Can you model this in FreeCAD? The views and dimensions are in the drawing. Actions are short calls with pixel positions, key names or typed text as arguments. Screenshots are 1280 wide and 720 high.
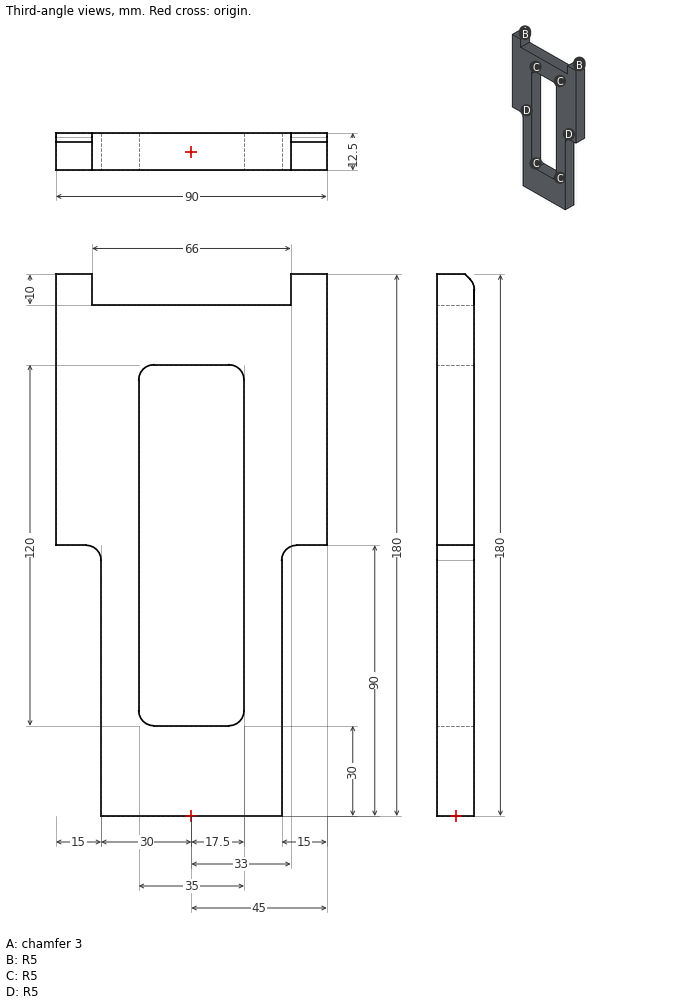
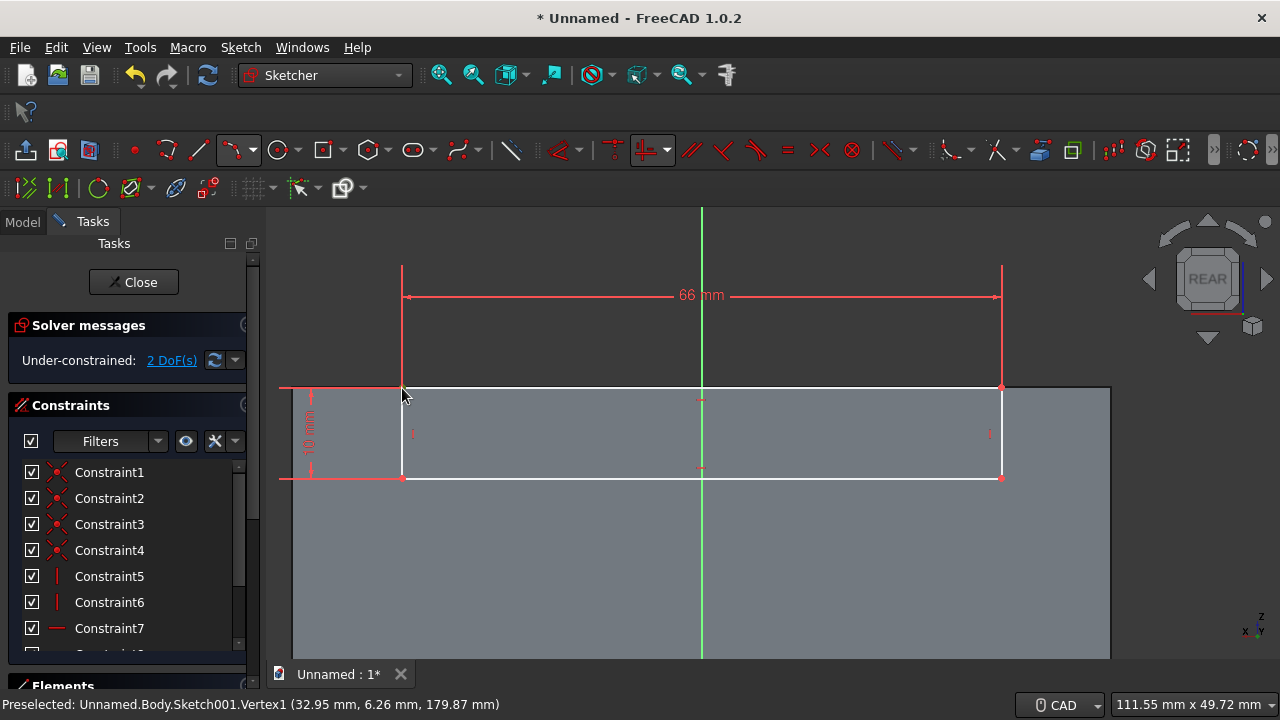
click(582, 150)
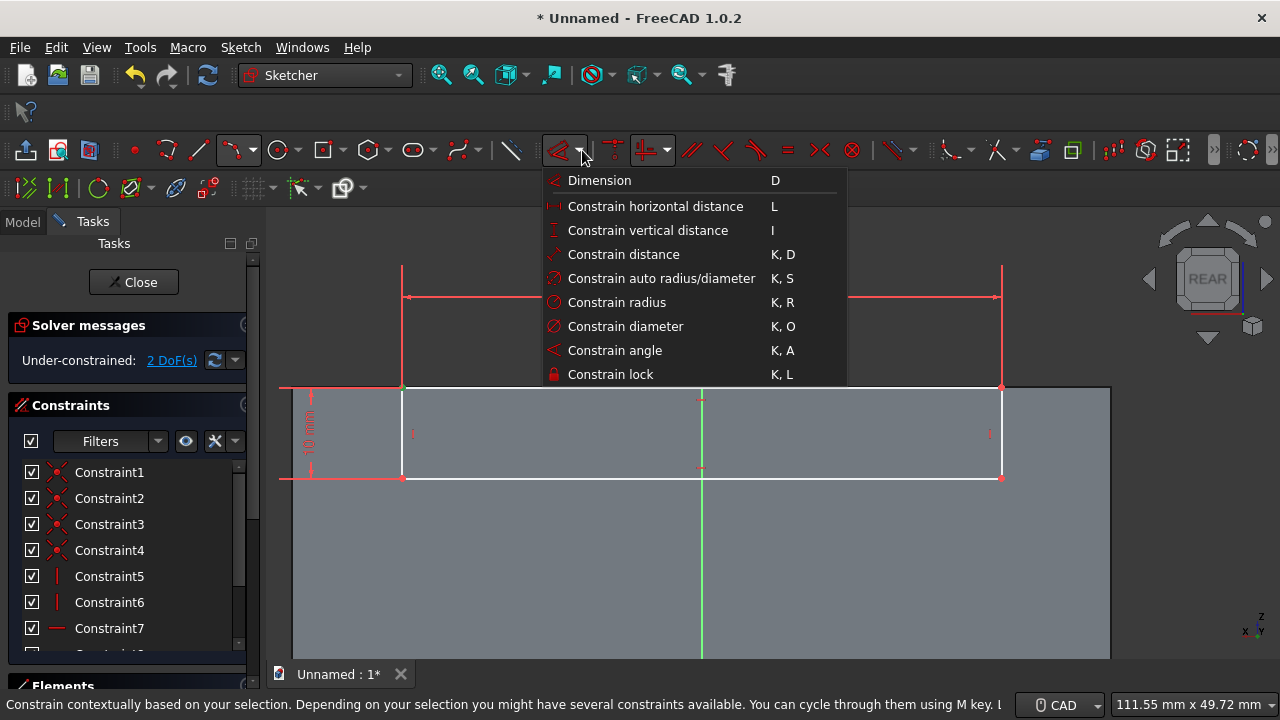
click(695, 206)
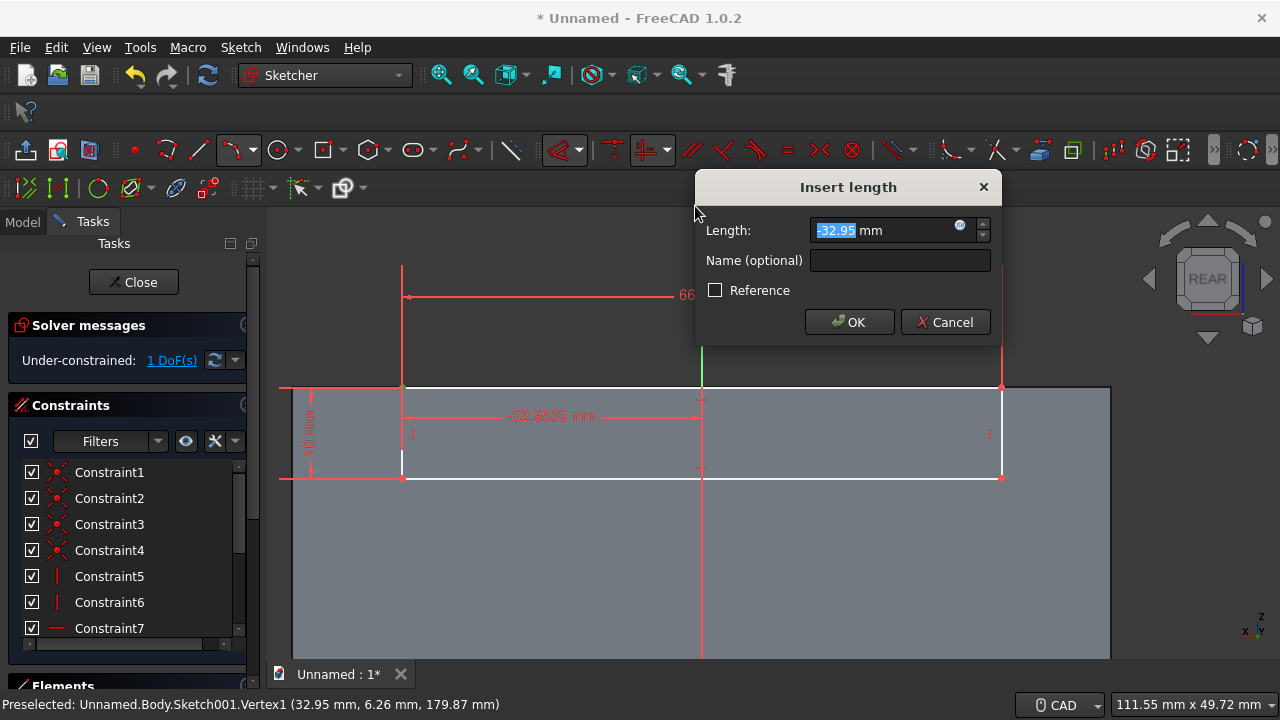
text(-33)
key(Return)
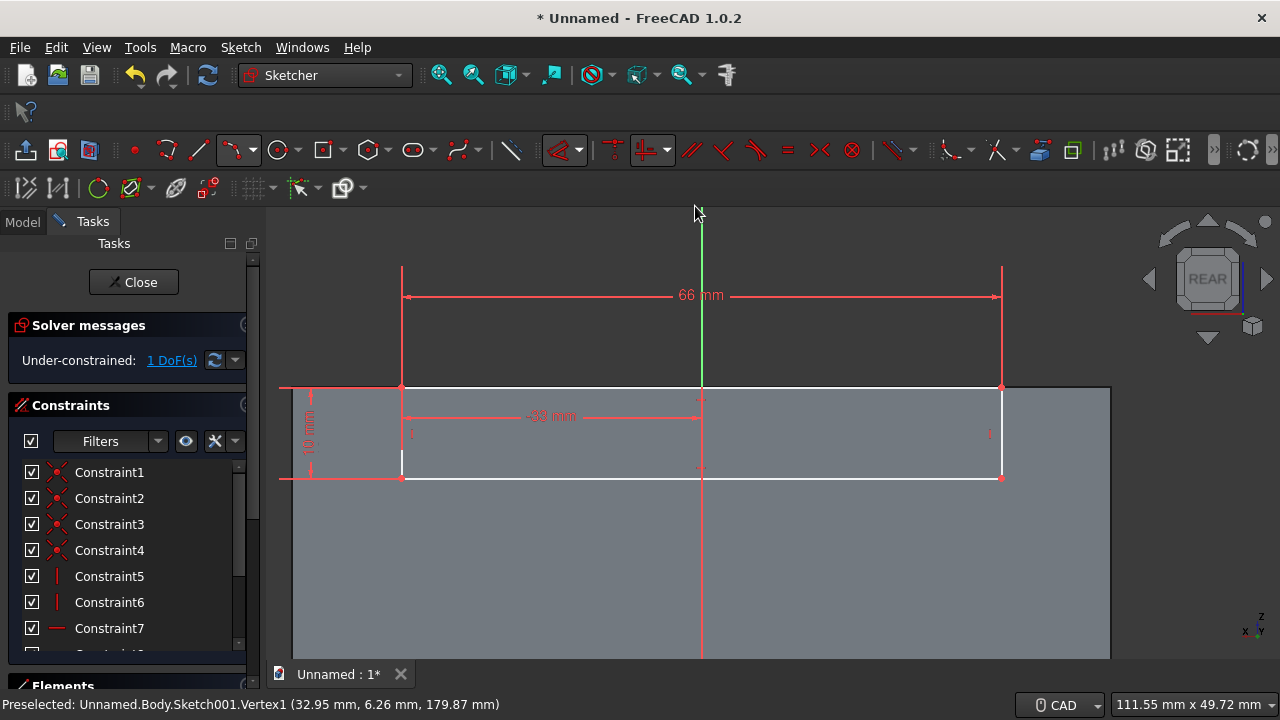
click(402, 388)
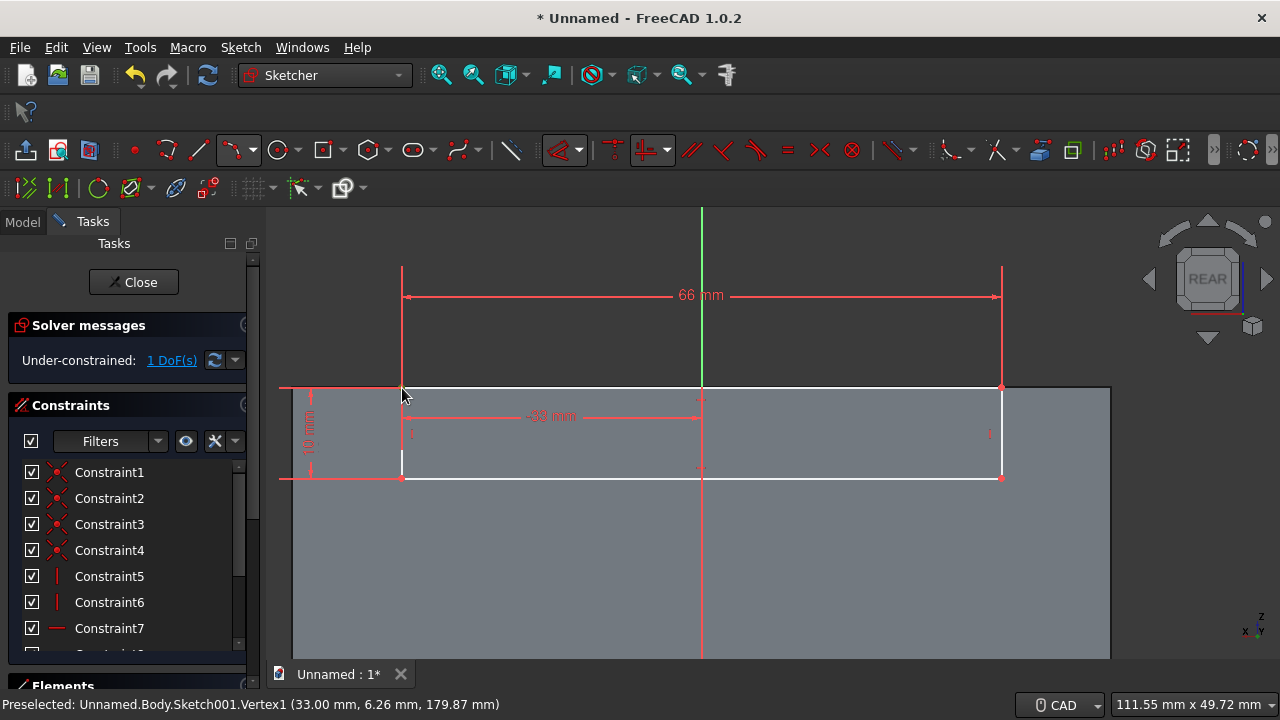
click(582, 150)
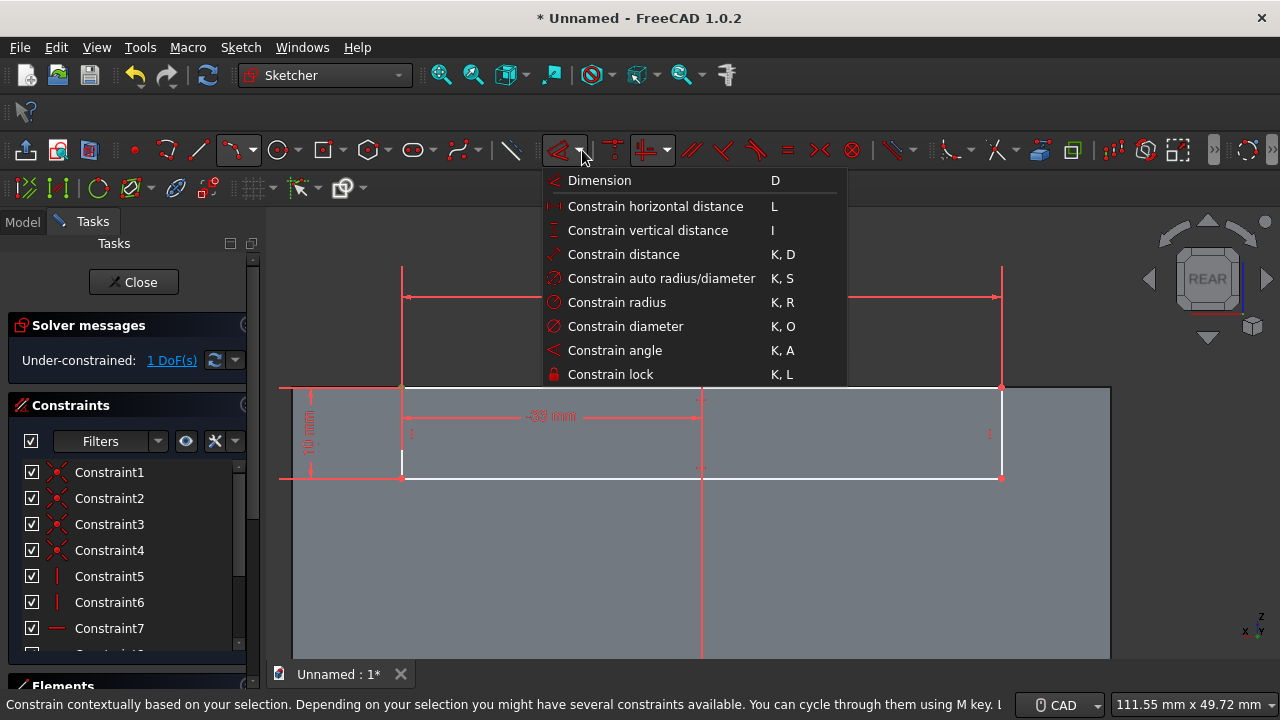
click(695, 230)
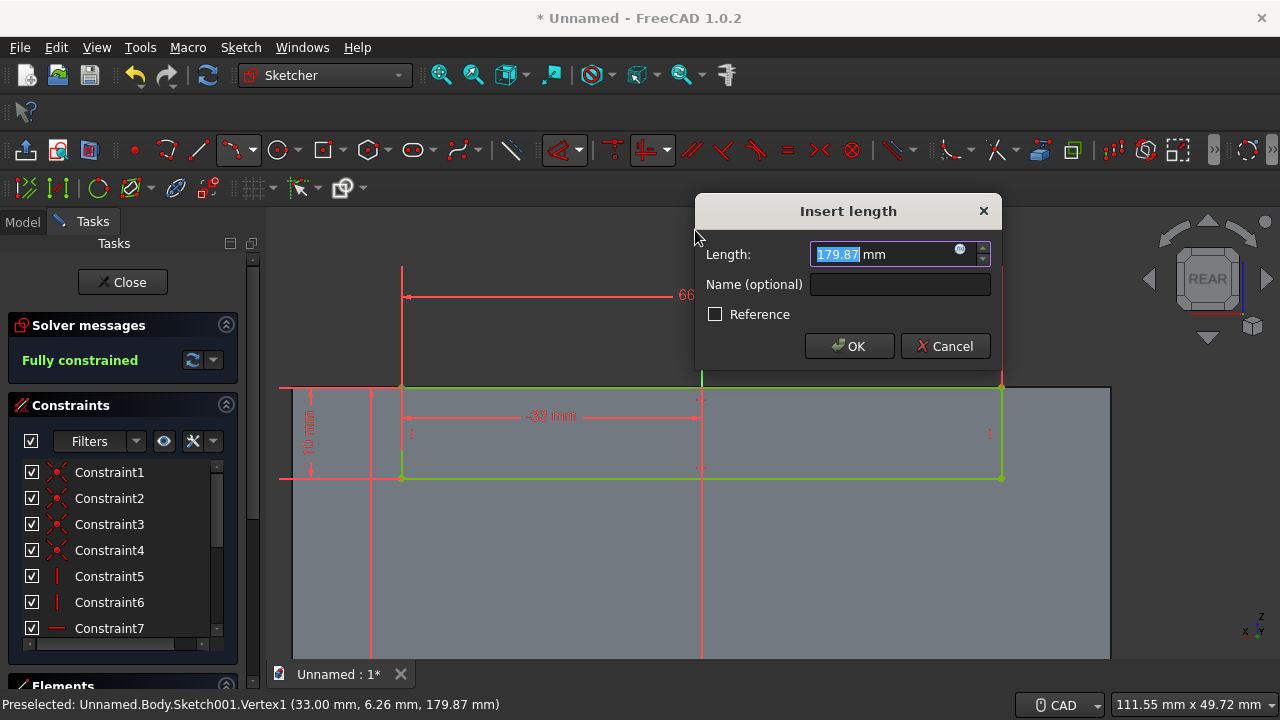
text(180)
key(Return)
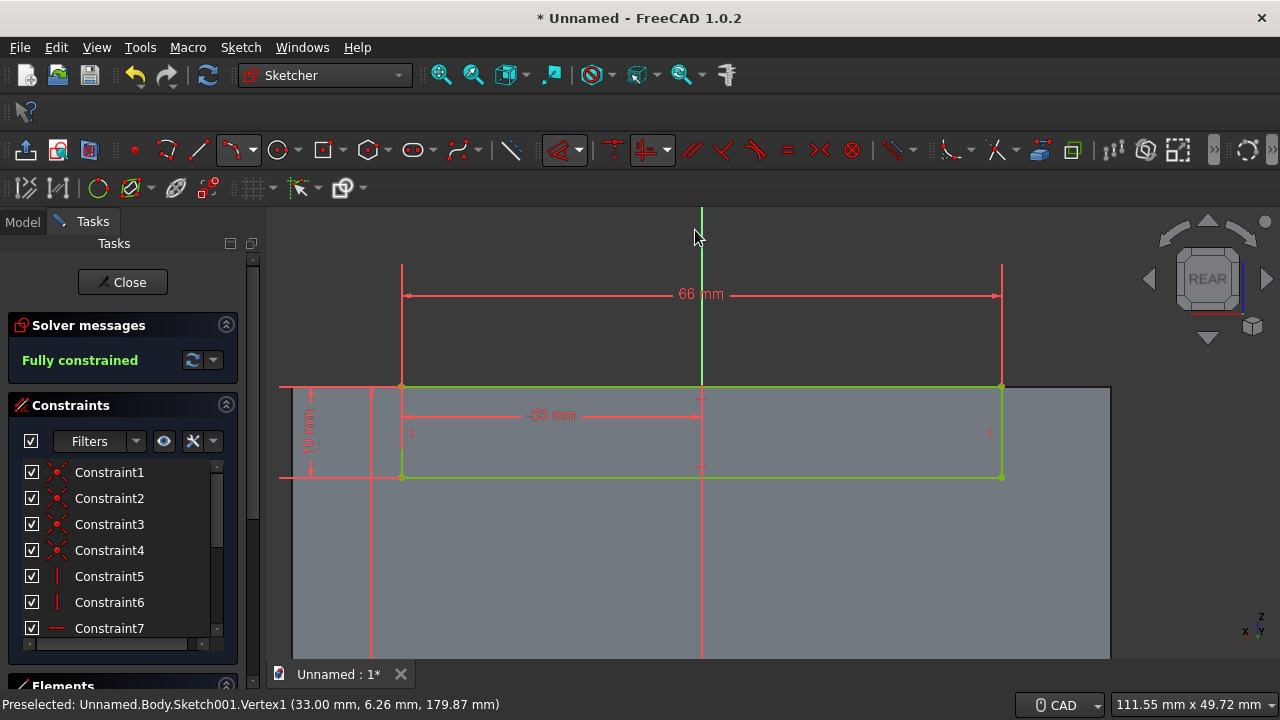
click(123, 282)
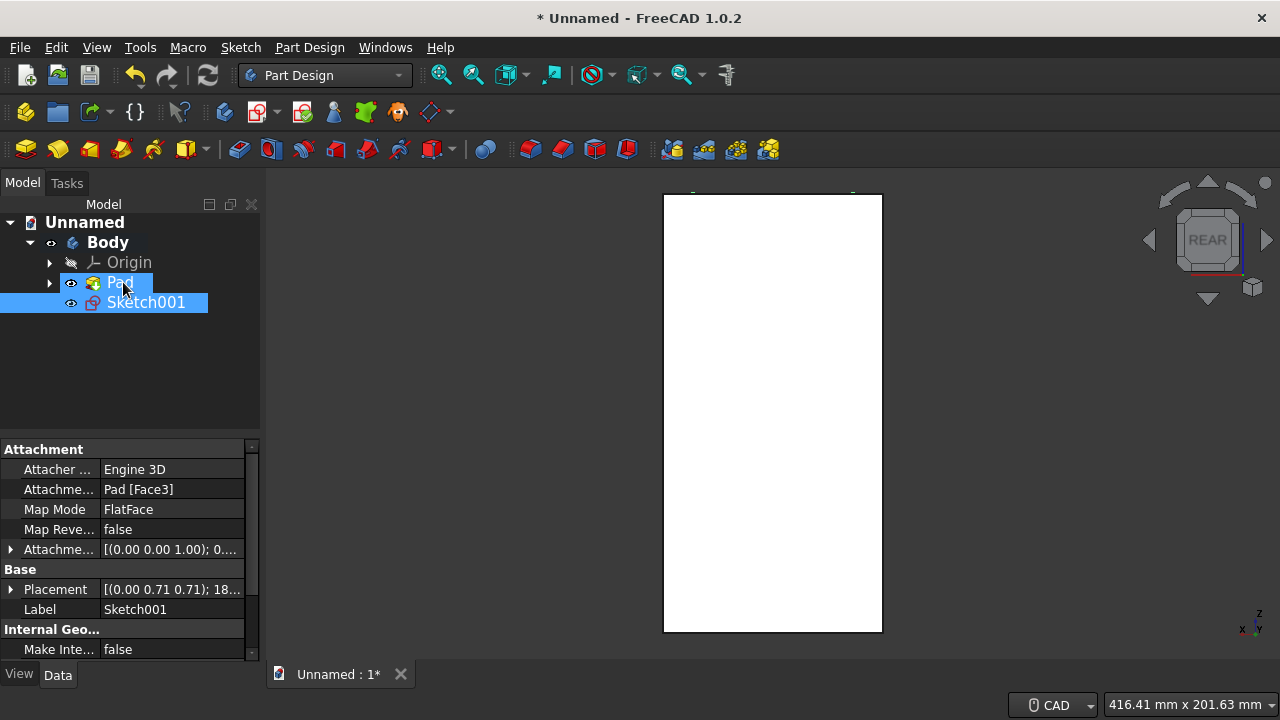
click(240, 150)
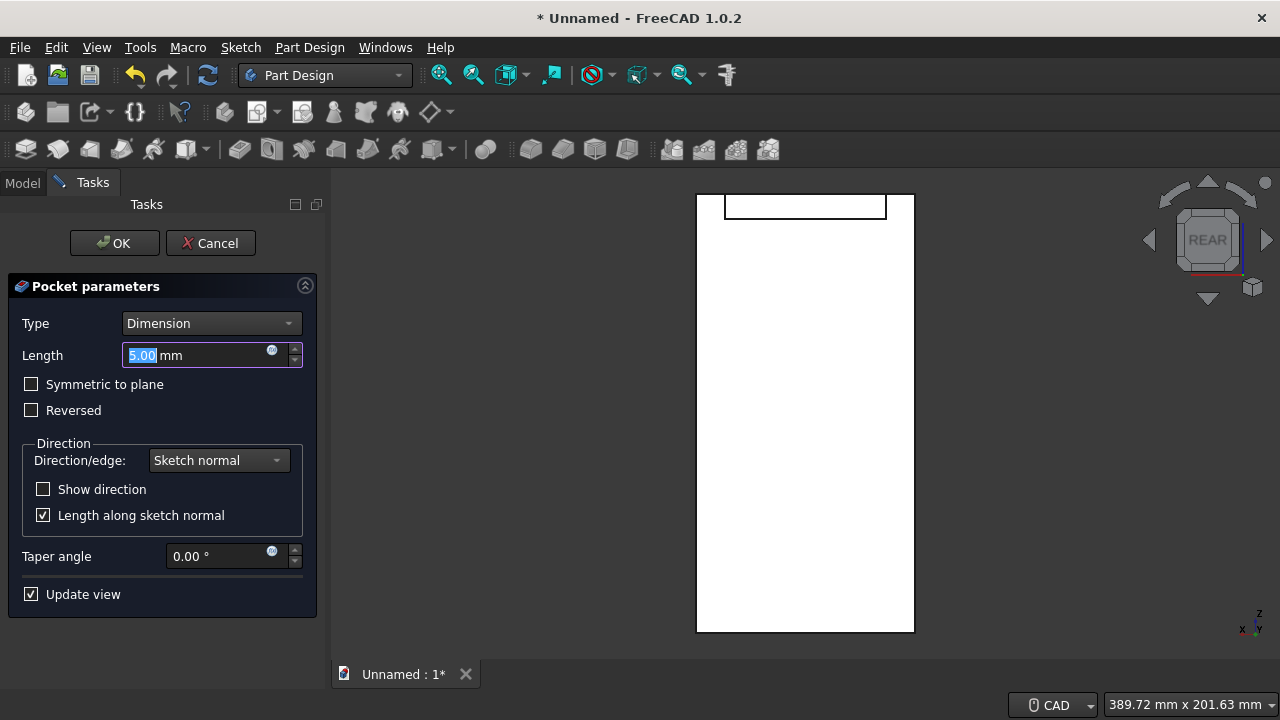
click(212, 324)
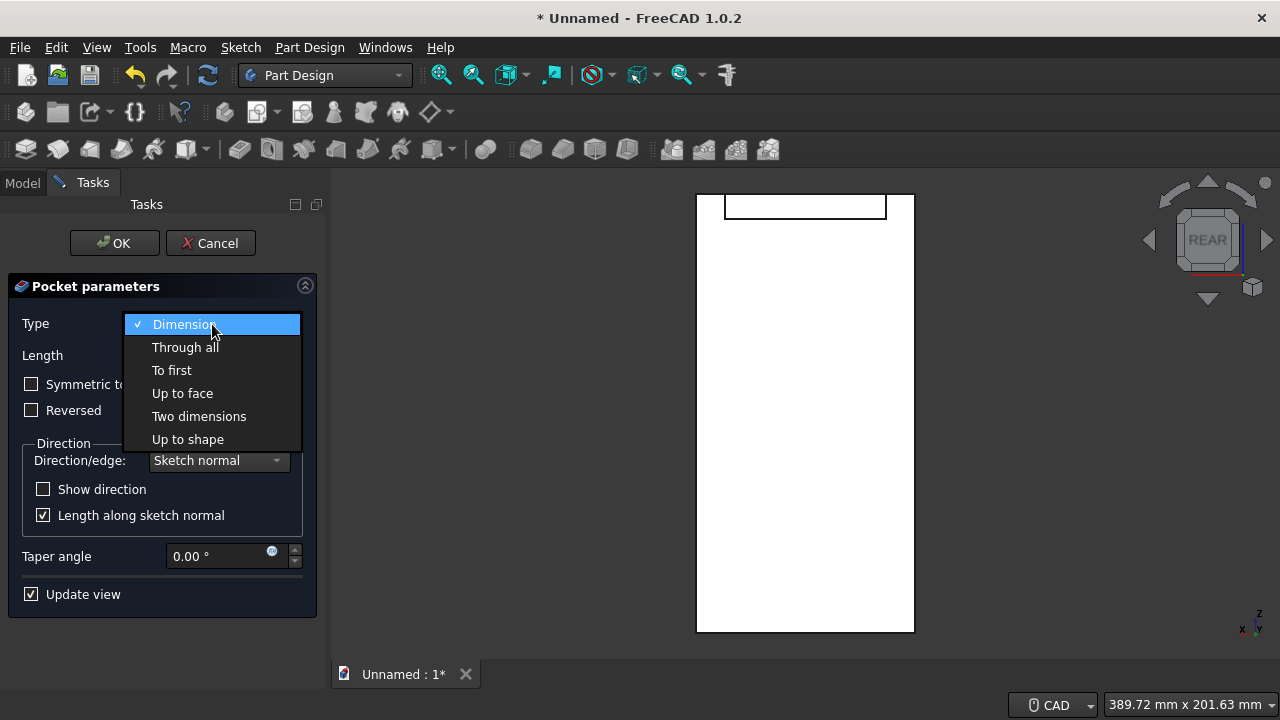
click(212, 348)